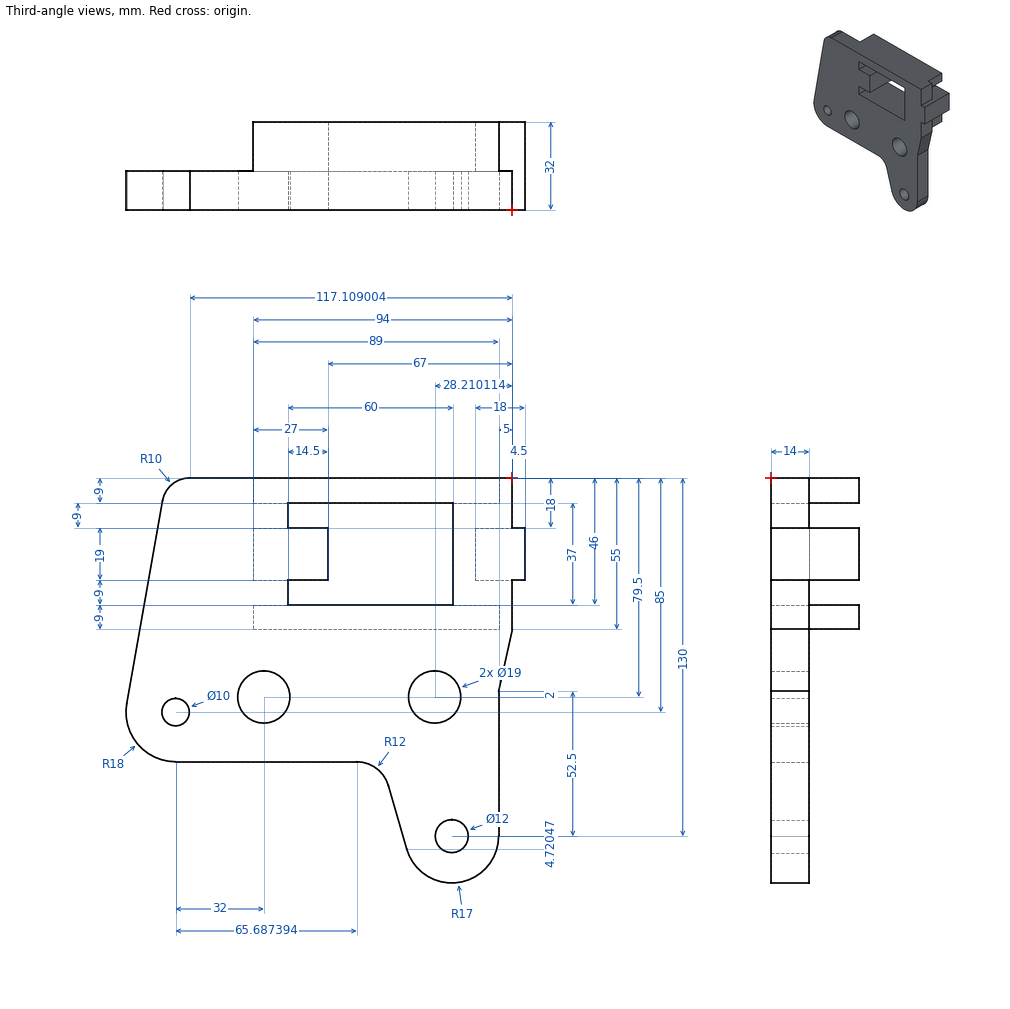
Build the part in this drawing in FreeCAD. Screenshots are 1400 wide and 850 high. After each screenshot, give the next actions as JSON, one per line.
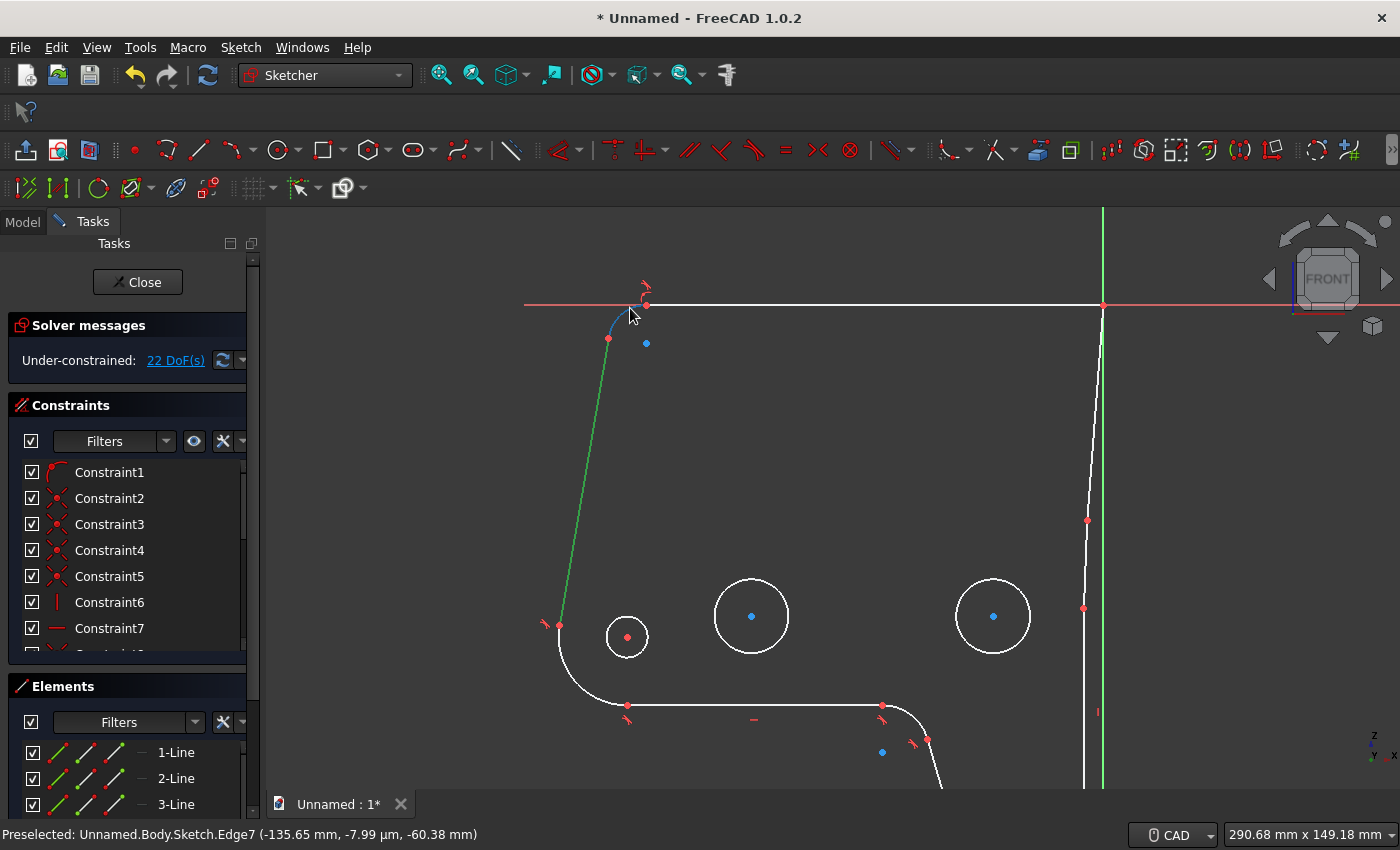
{"action": "left_click", "coordinate": [631, 309]}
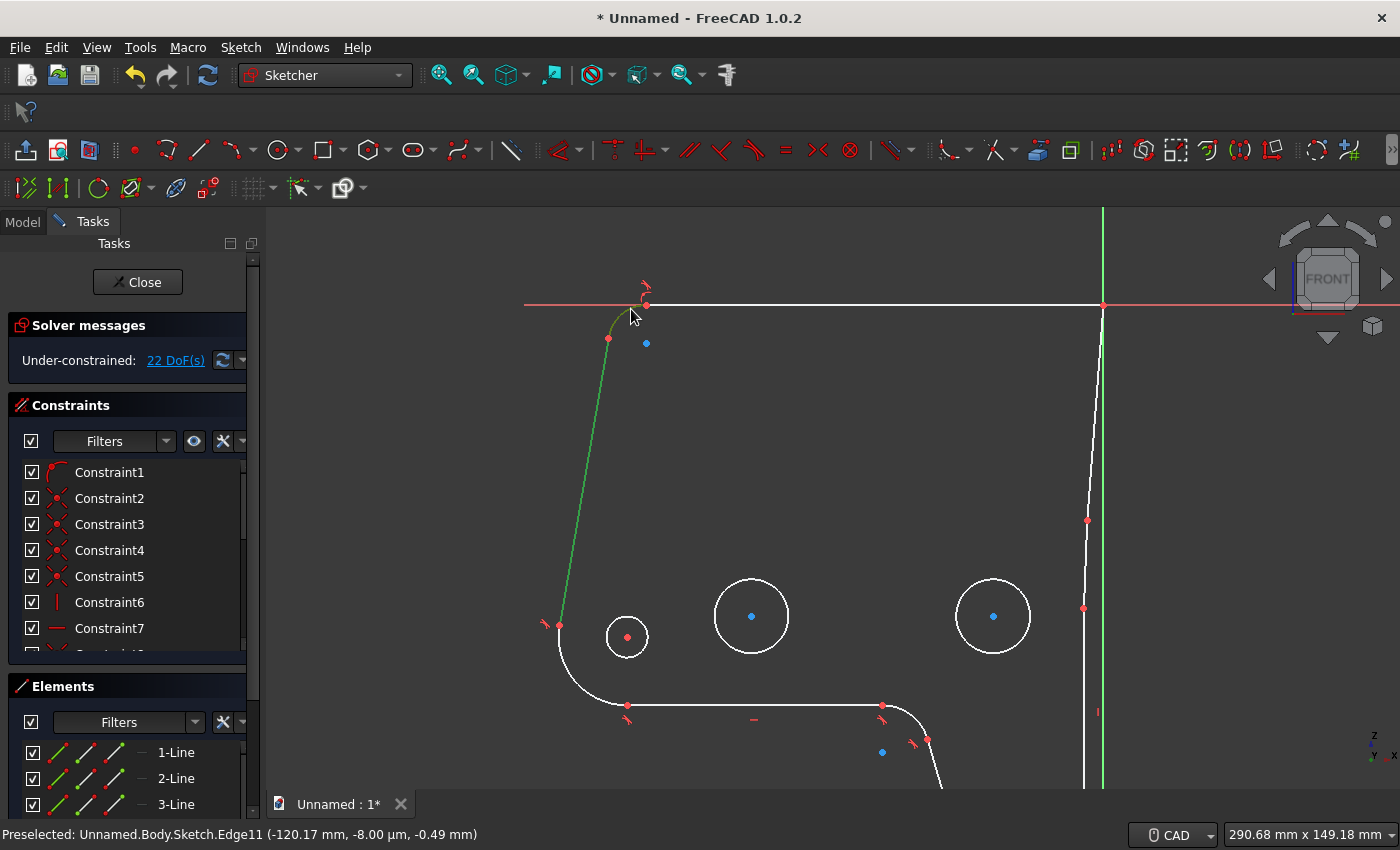
{"action": "left_click", "coordinate": [754, 150]}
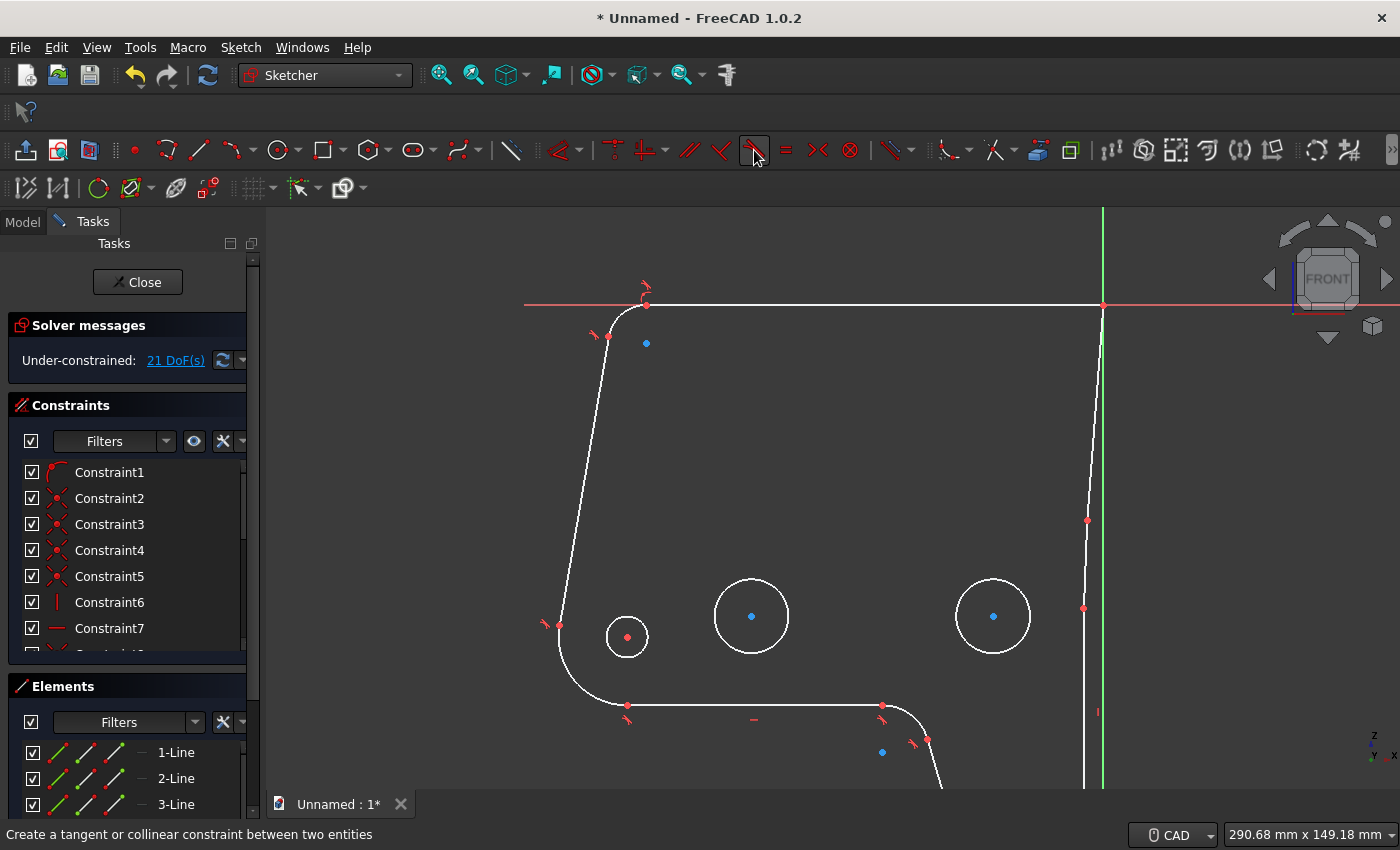
{"action": "left_click", "coordinate": [1092, 456]}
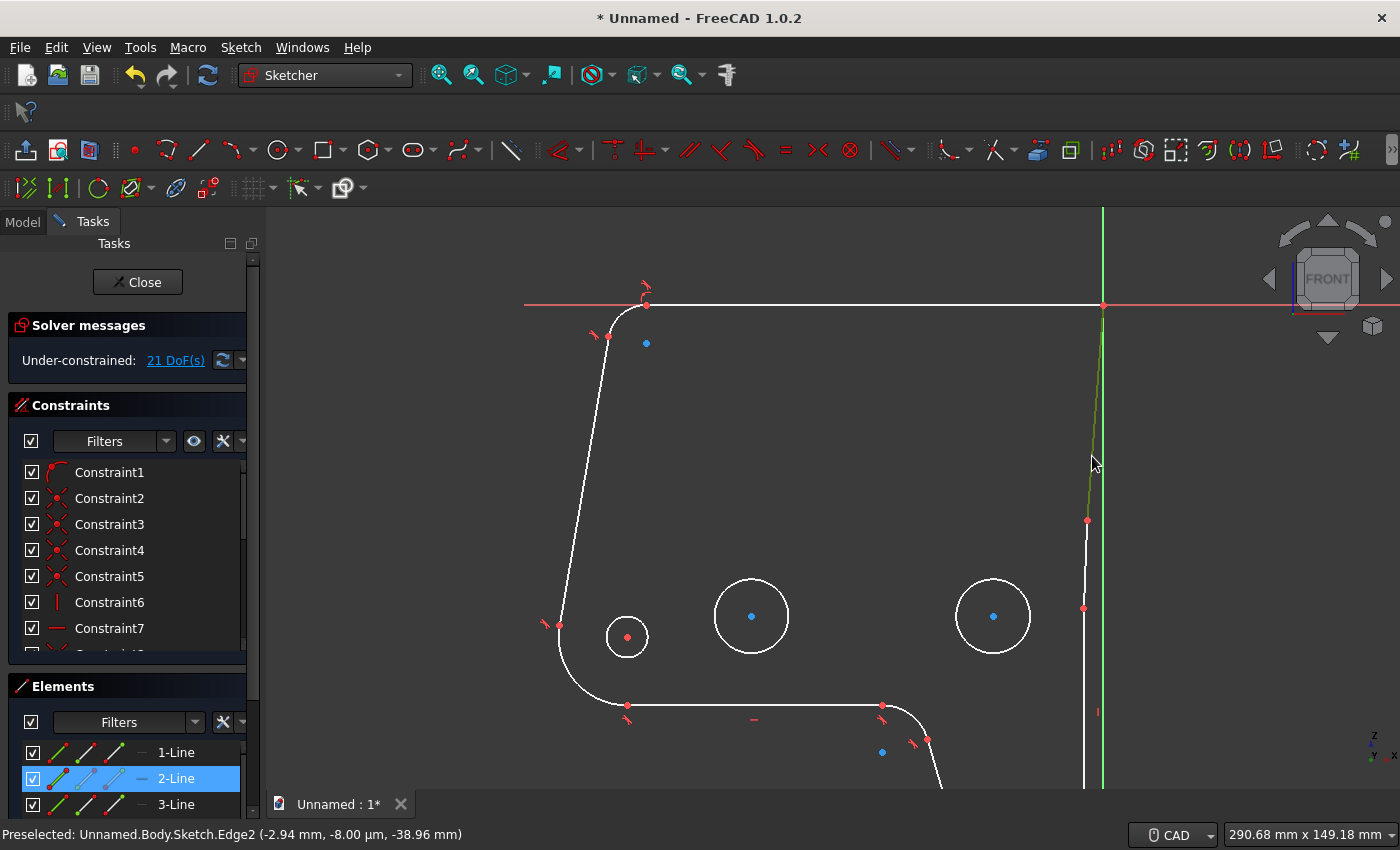
{"action": "key", "text": "v"}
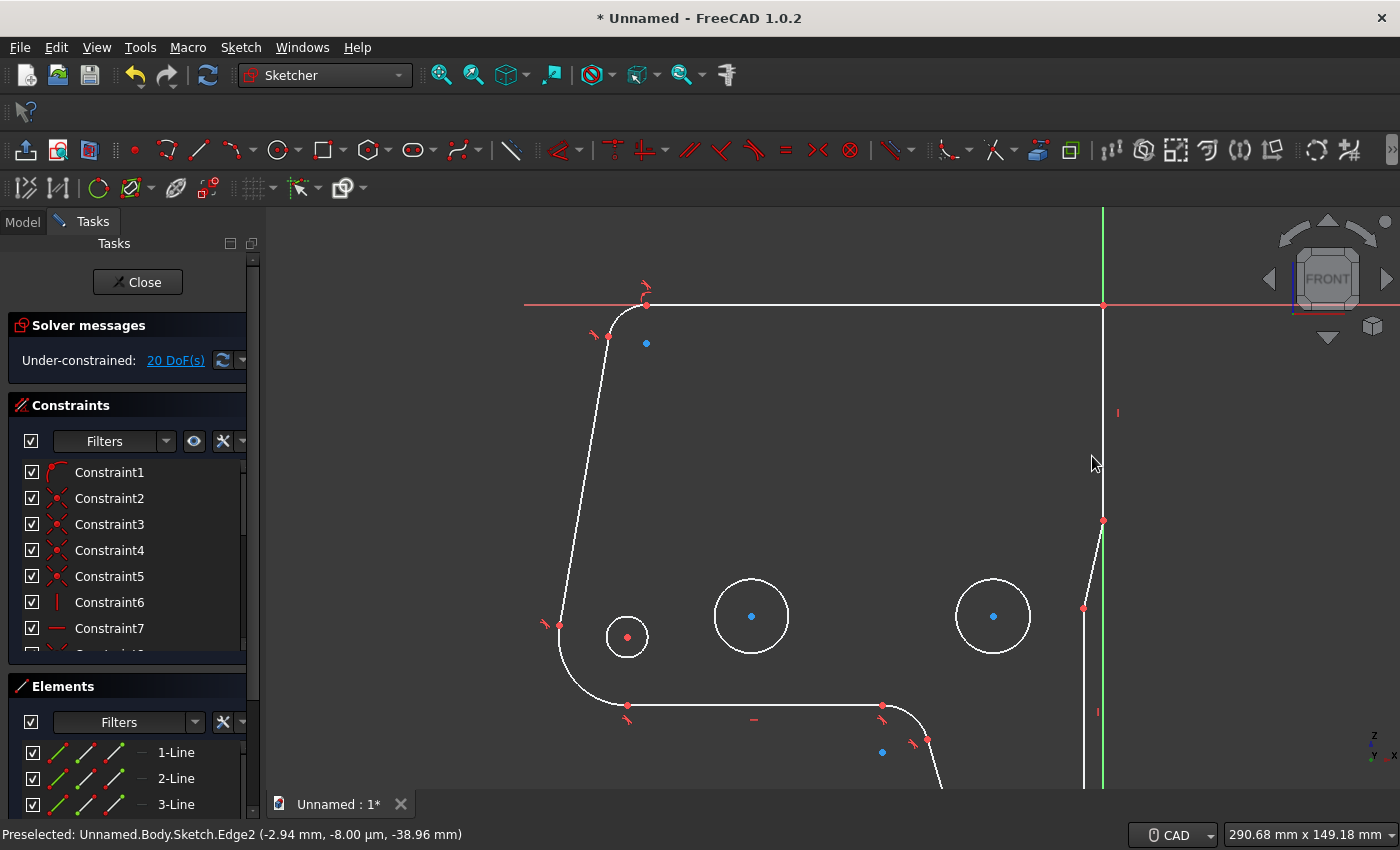
{"action": "left_click", "coordinate": [1019, 590]}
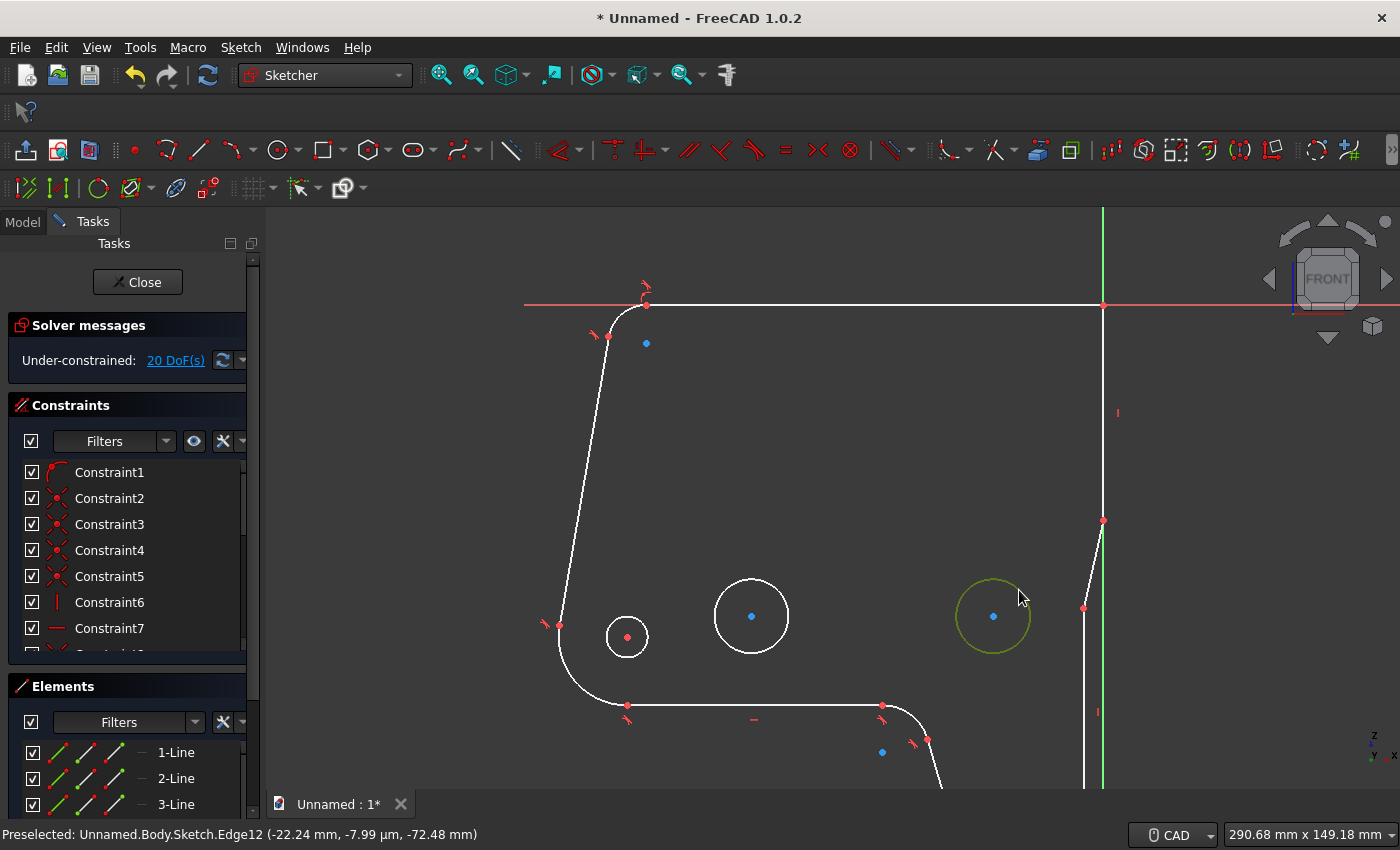
{"action": "left_click", "coordinate": [778, 590]}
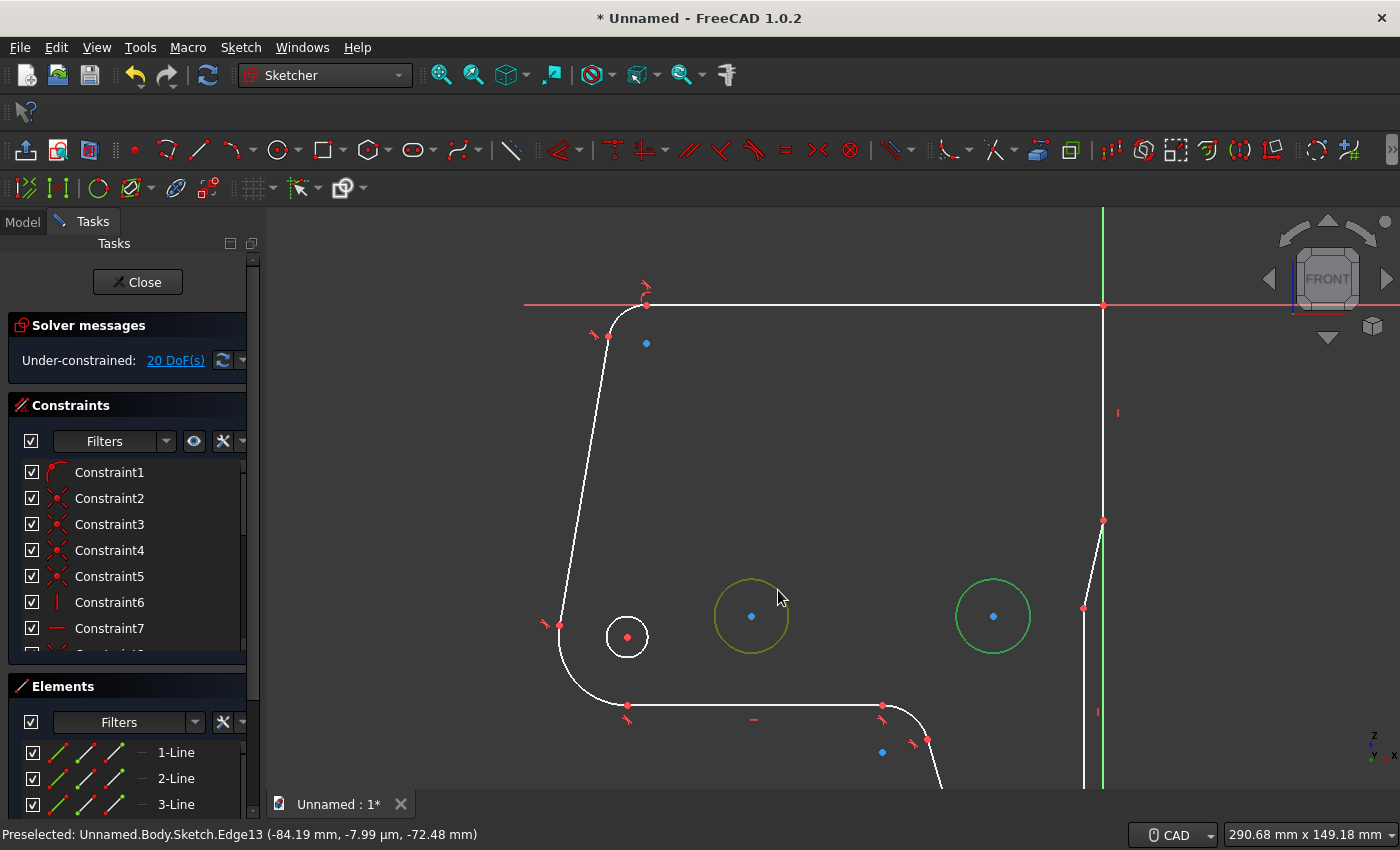
{"action": "key", "text": "e"}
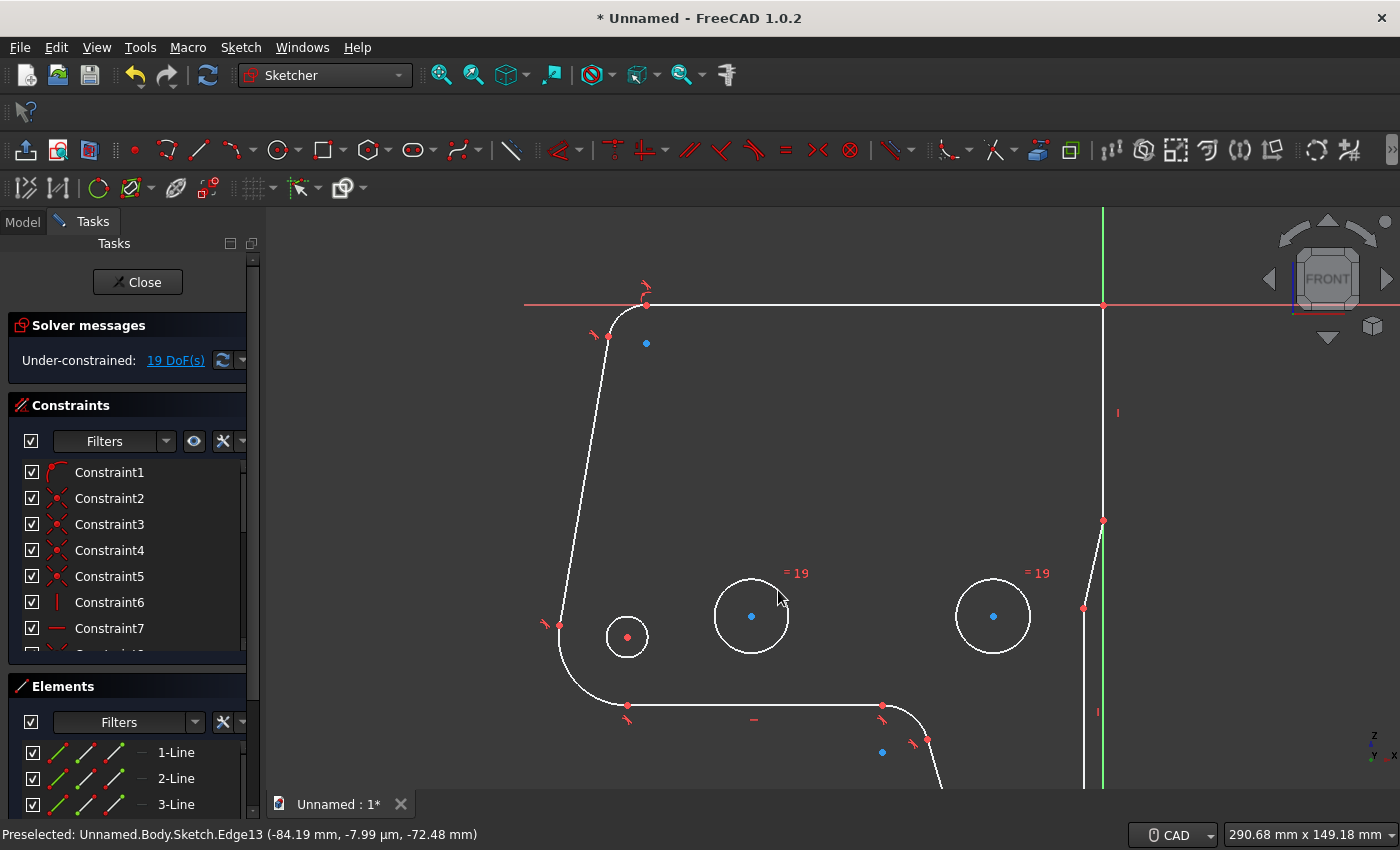
{"action": "left_click", "coordinate": [558, 150]}